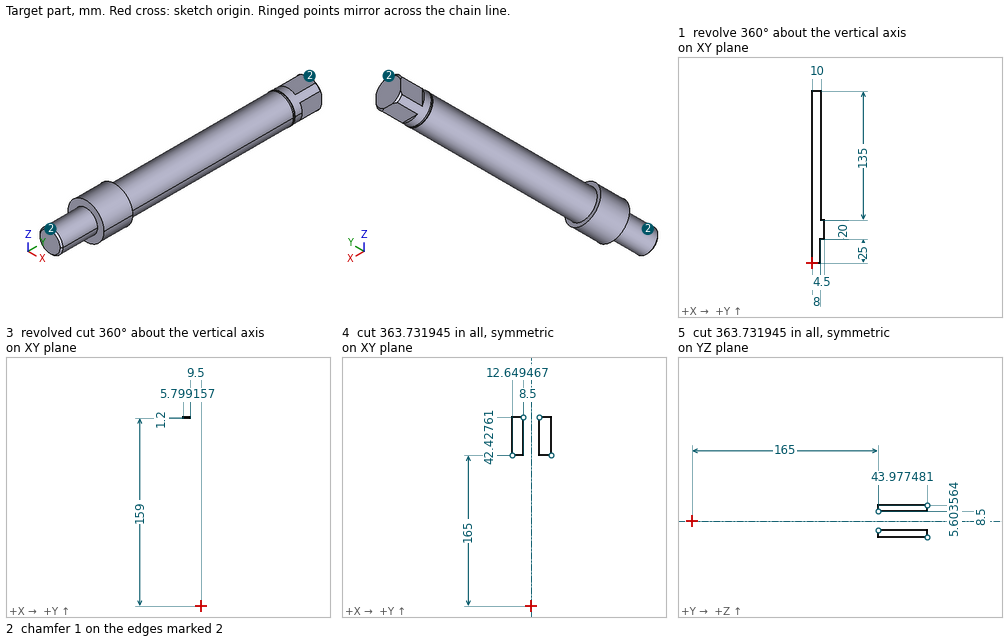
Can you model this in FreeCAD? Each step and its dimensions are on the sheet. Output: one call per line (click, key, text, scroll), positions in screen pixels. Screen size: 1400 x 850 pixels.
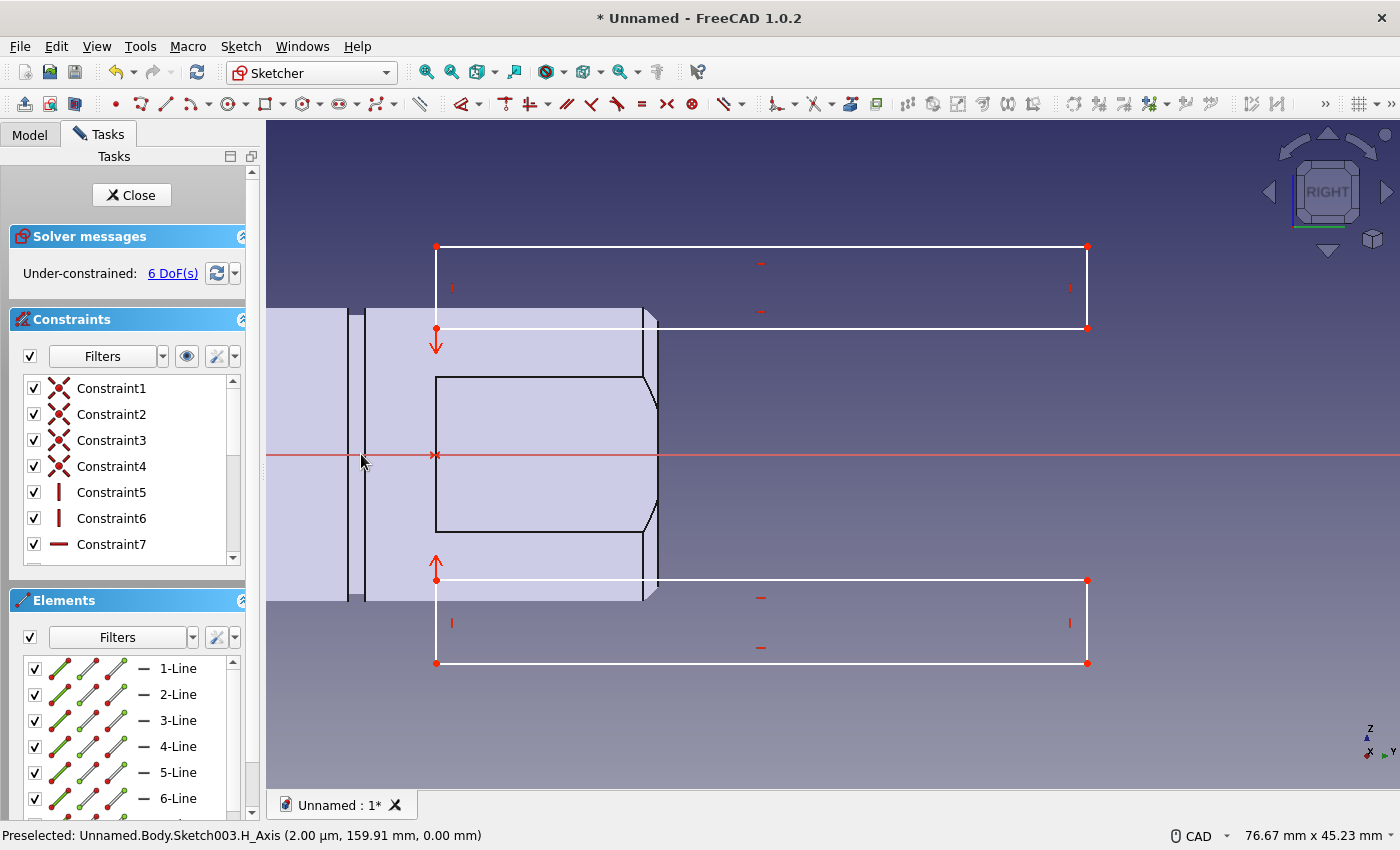
click(1087, 247)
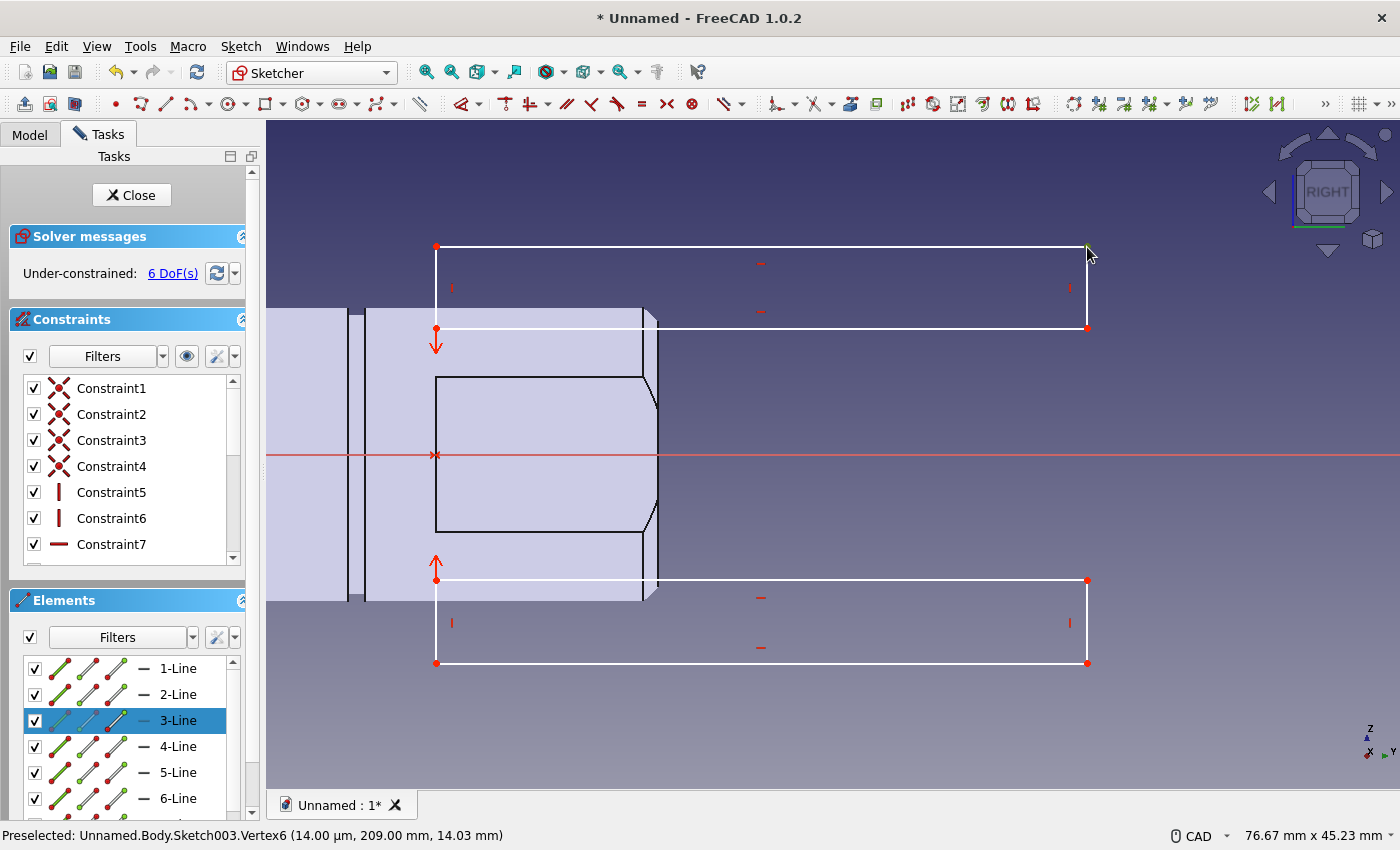
click(1087, 664)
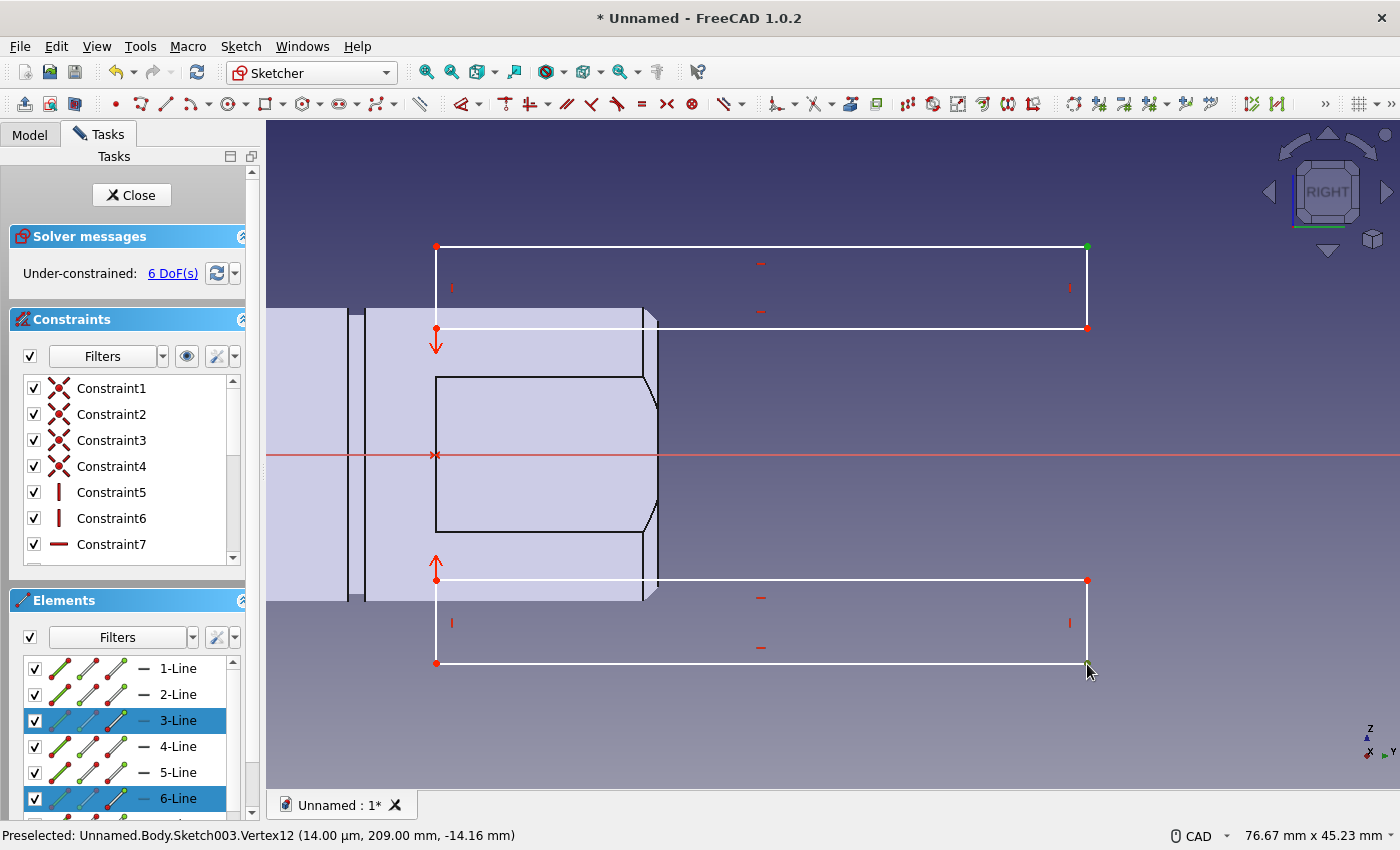
click(361, 454)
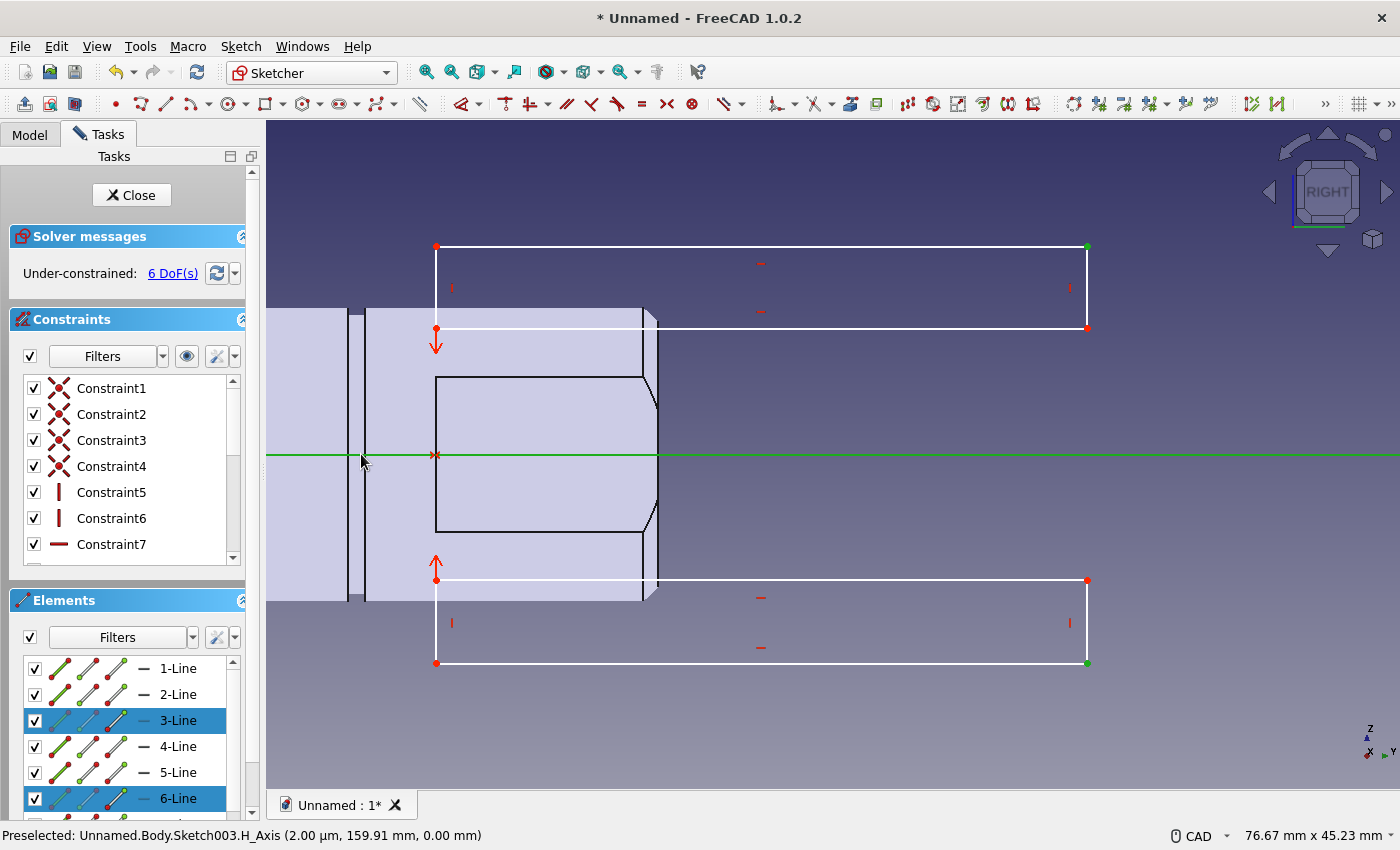
key(s)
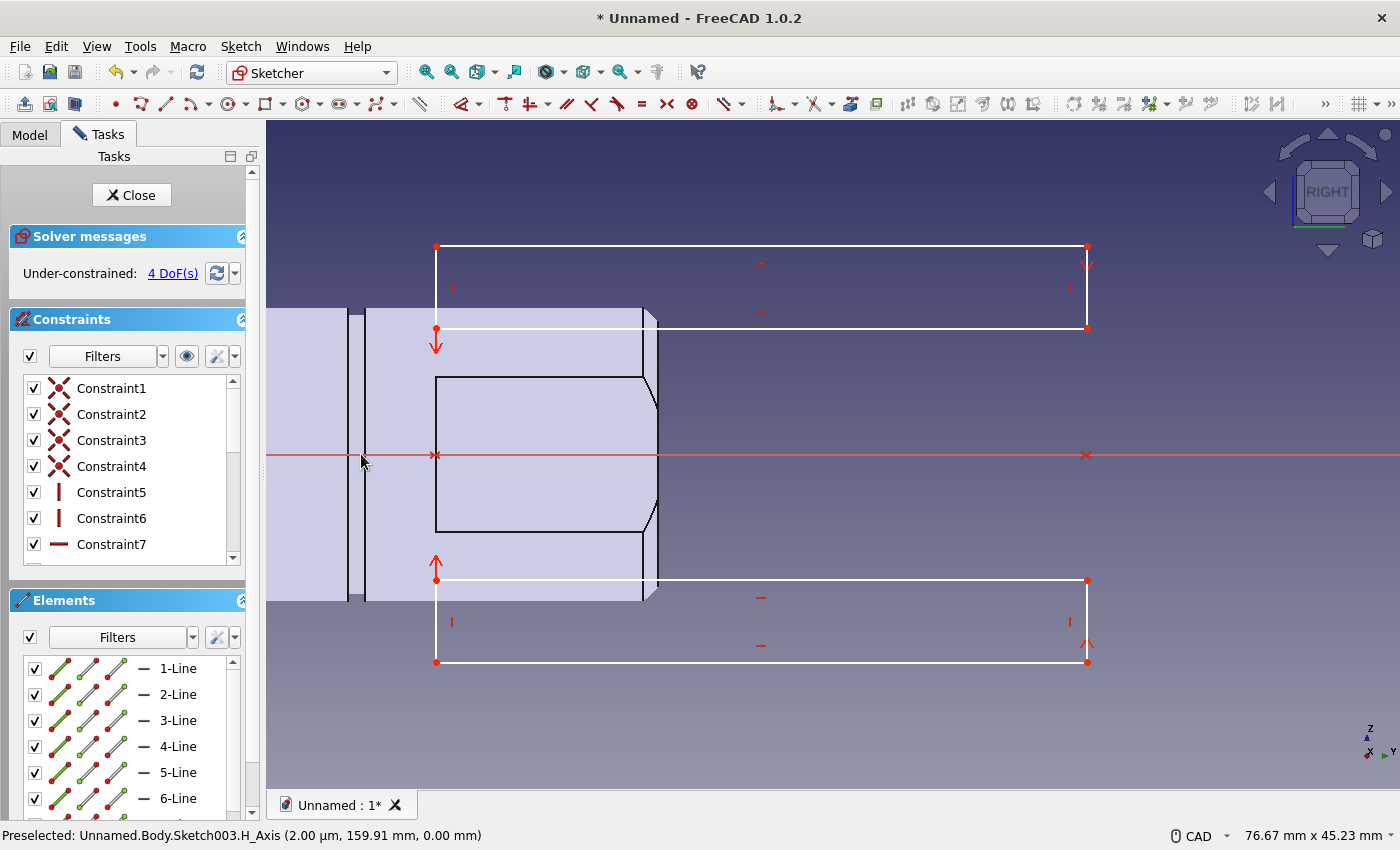
key(d)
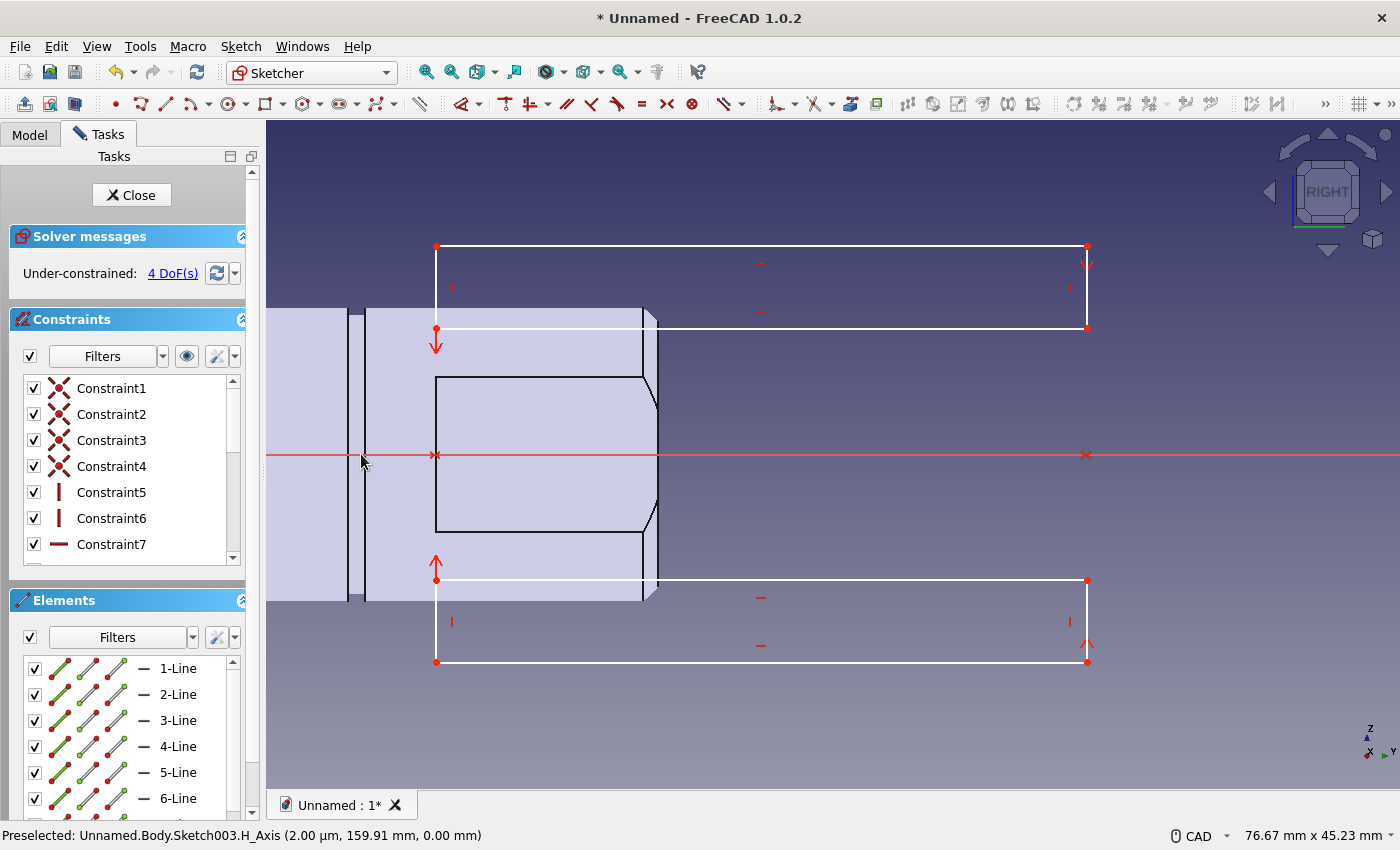
click(436, 246)
click(365, 212)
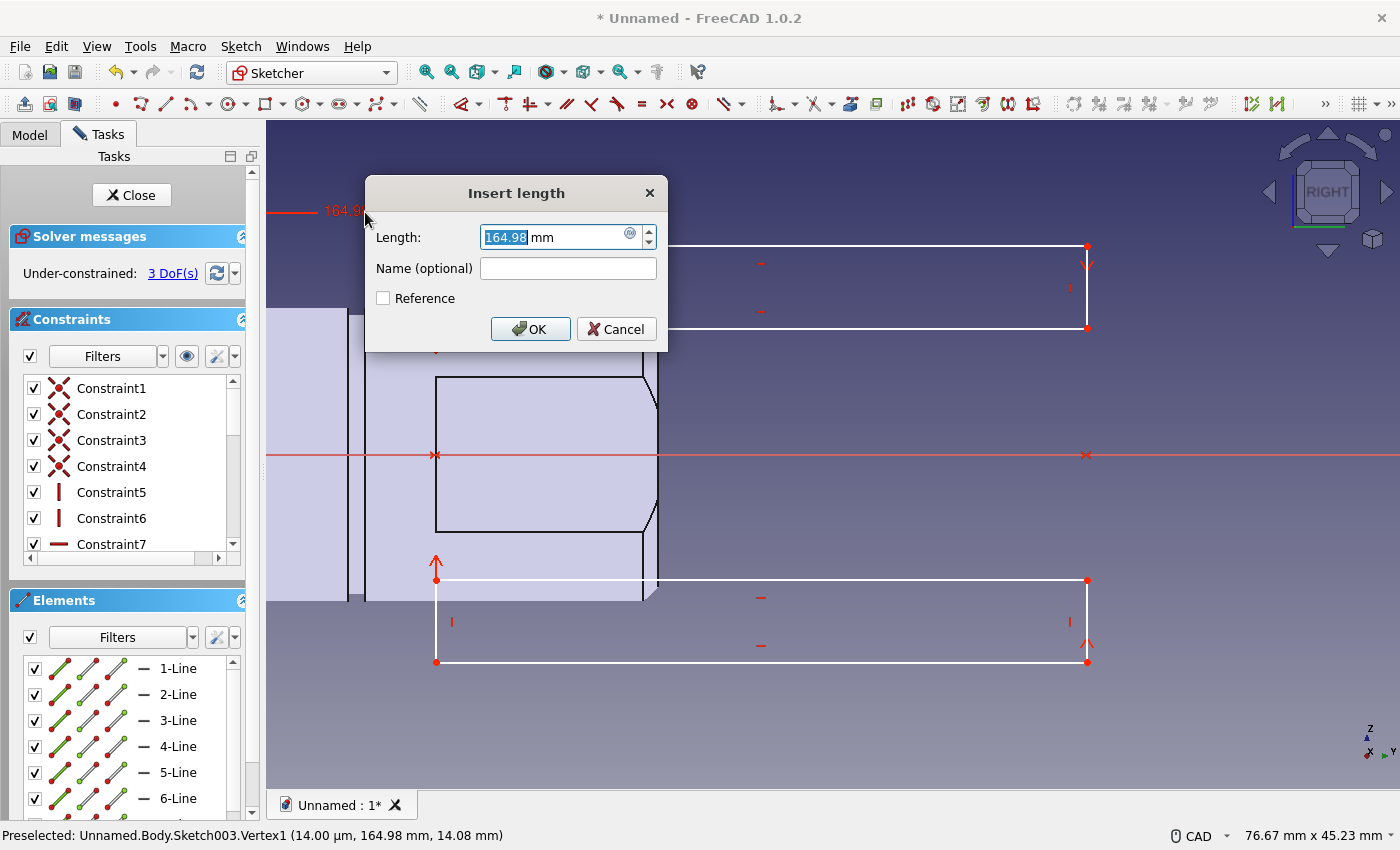
text(165)
key(Return)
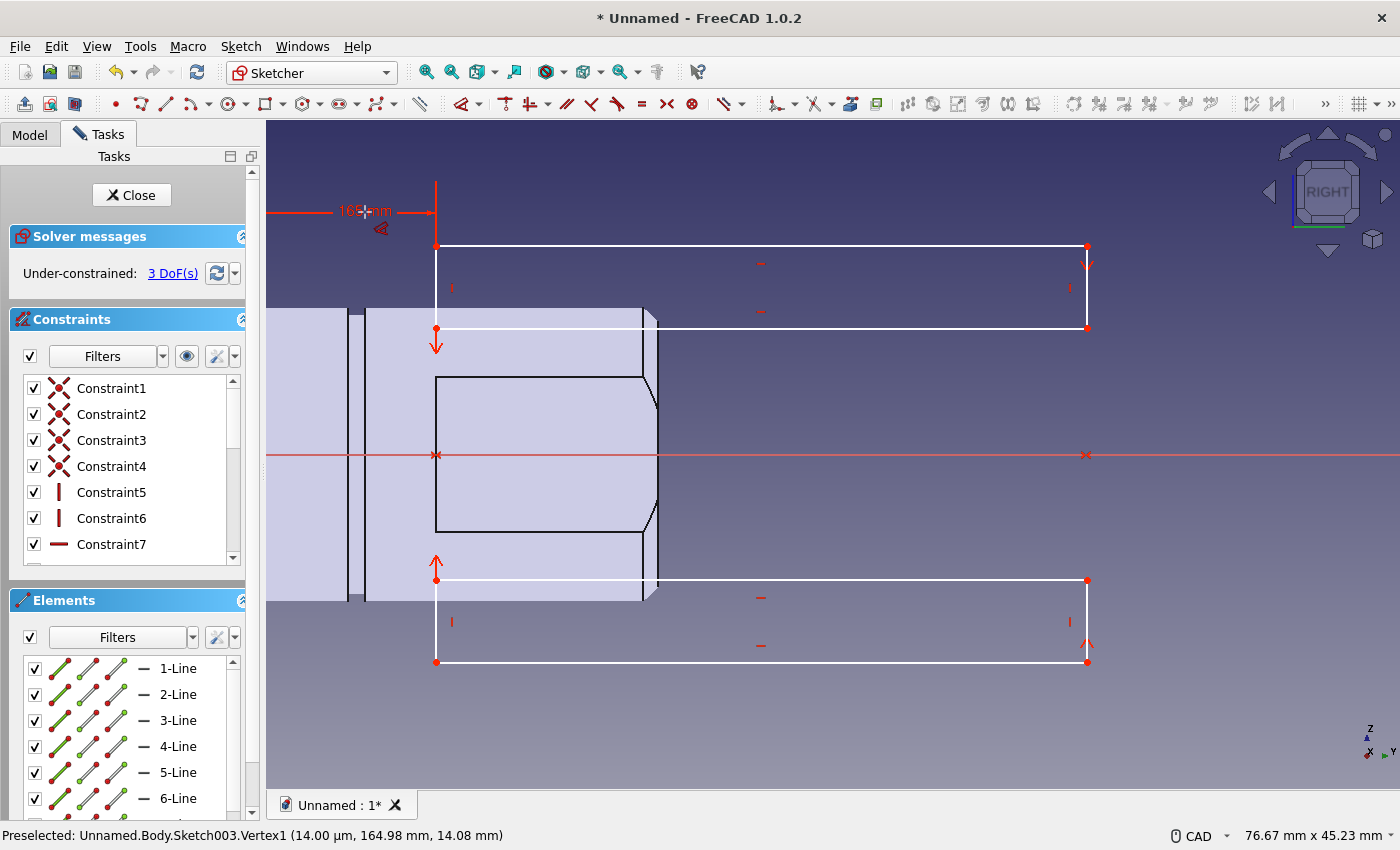
click(436, 329)
click(470, 392)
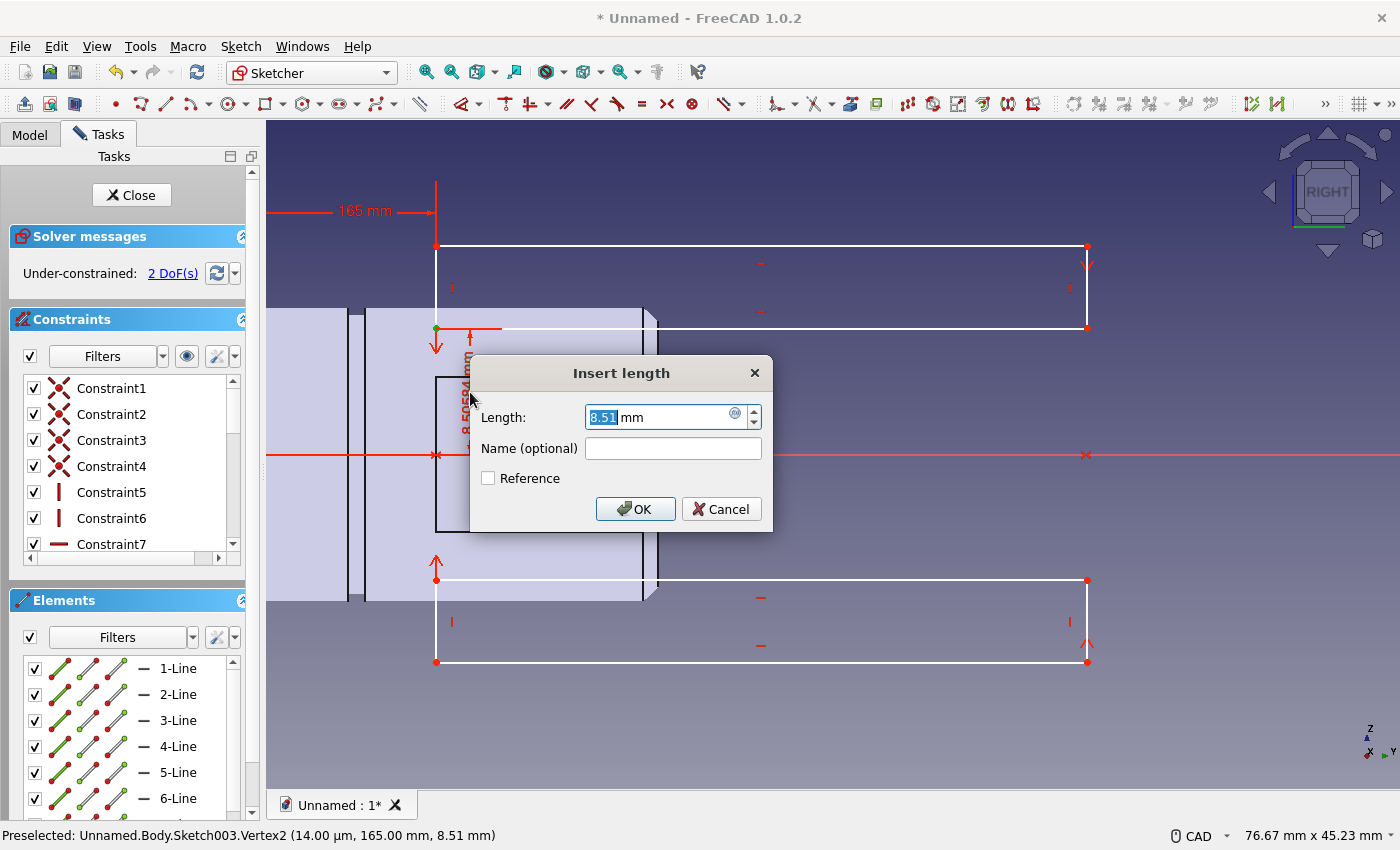
text(8.5)
key(Return)